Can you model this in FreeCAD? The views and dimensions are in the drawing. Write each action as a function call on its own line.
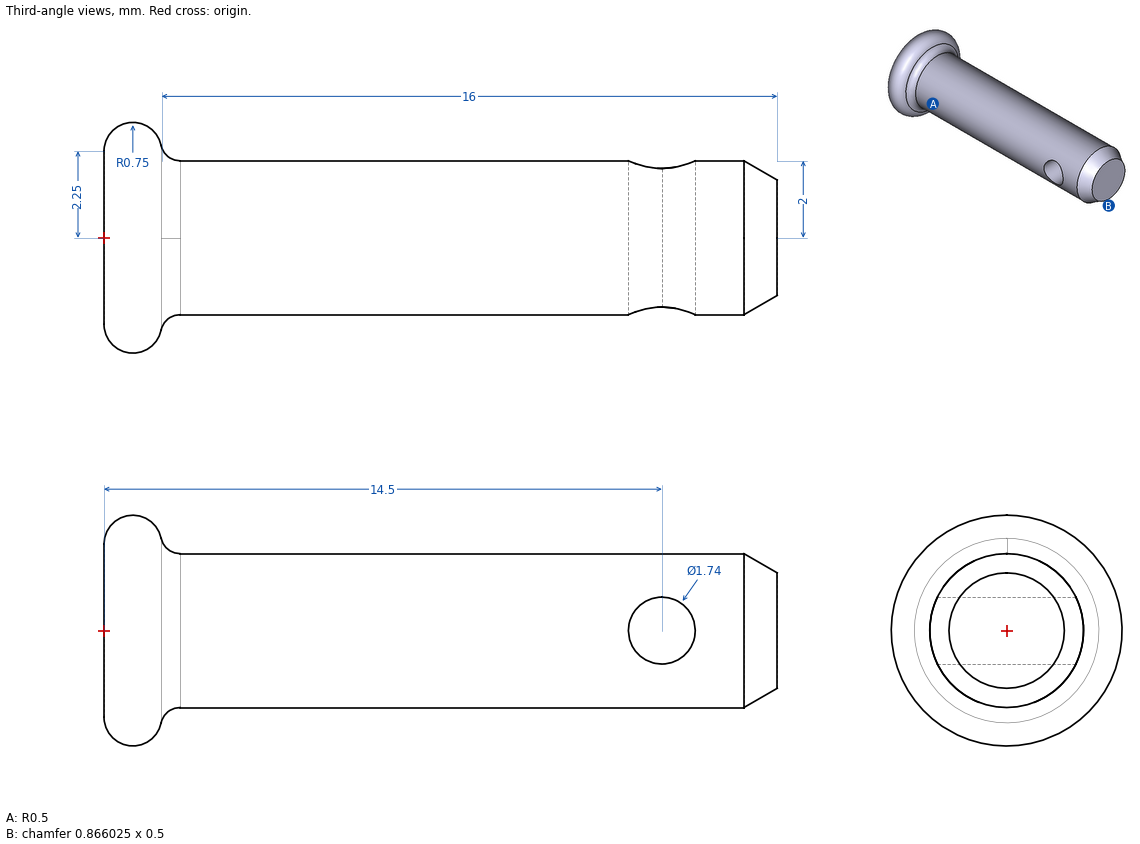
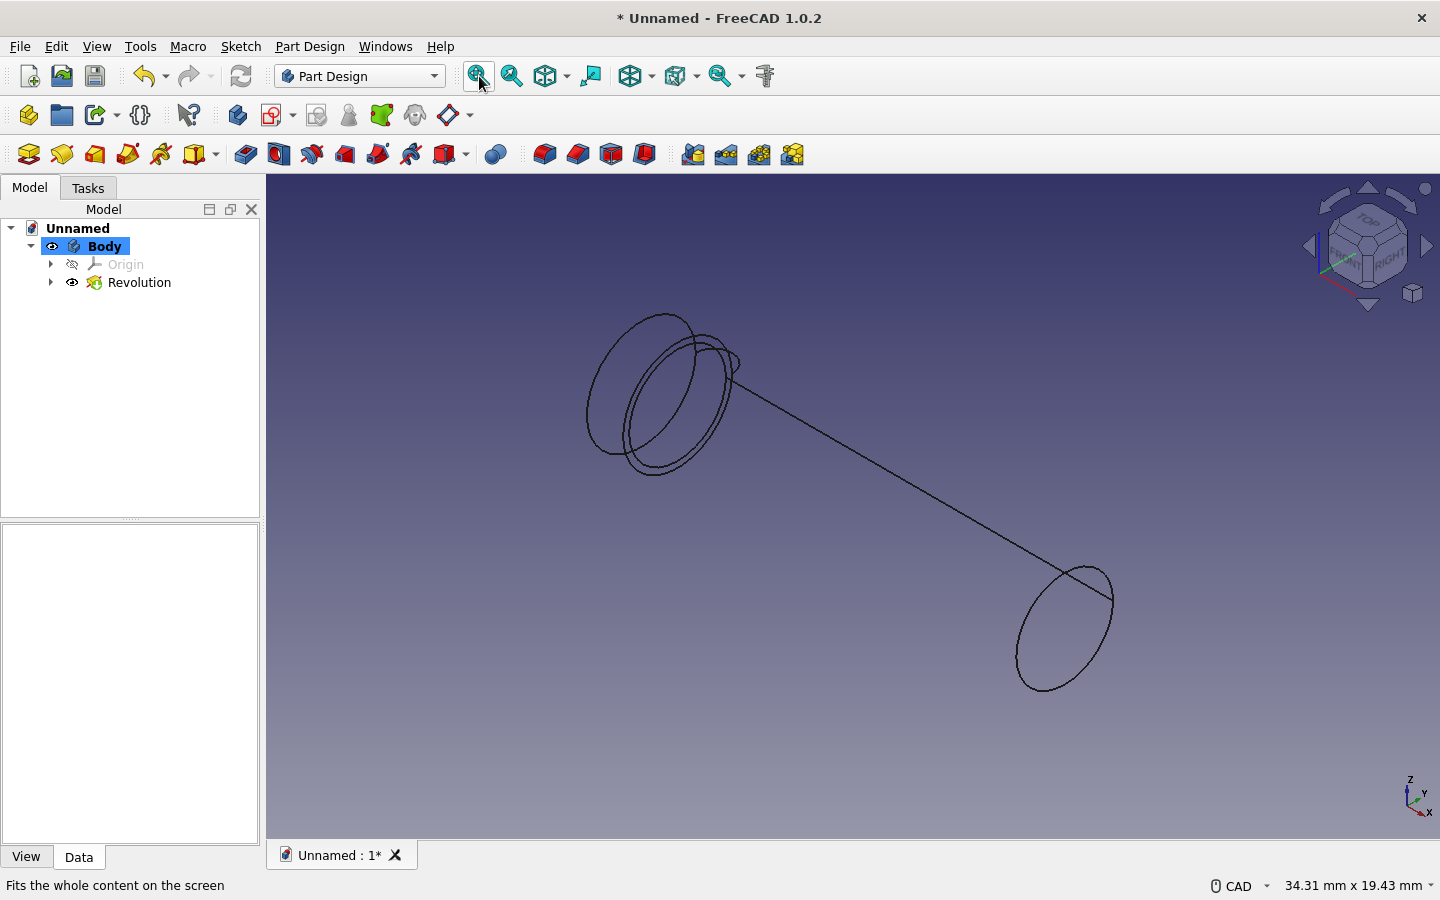
click(638, 460)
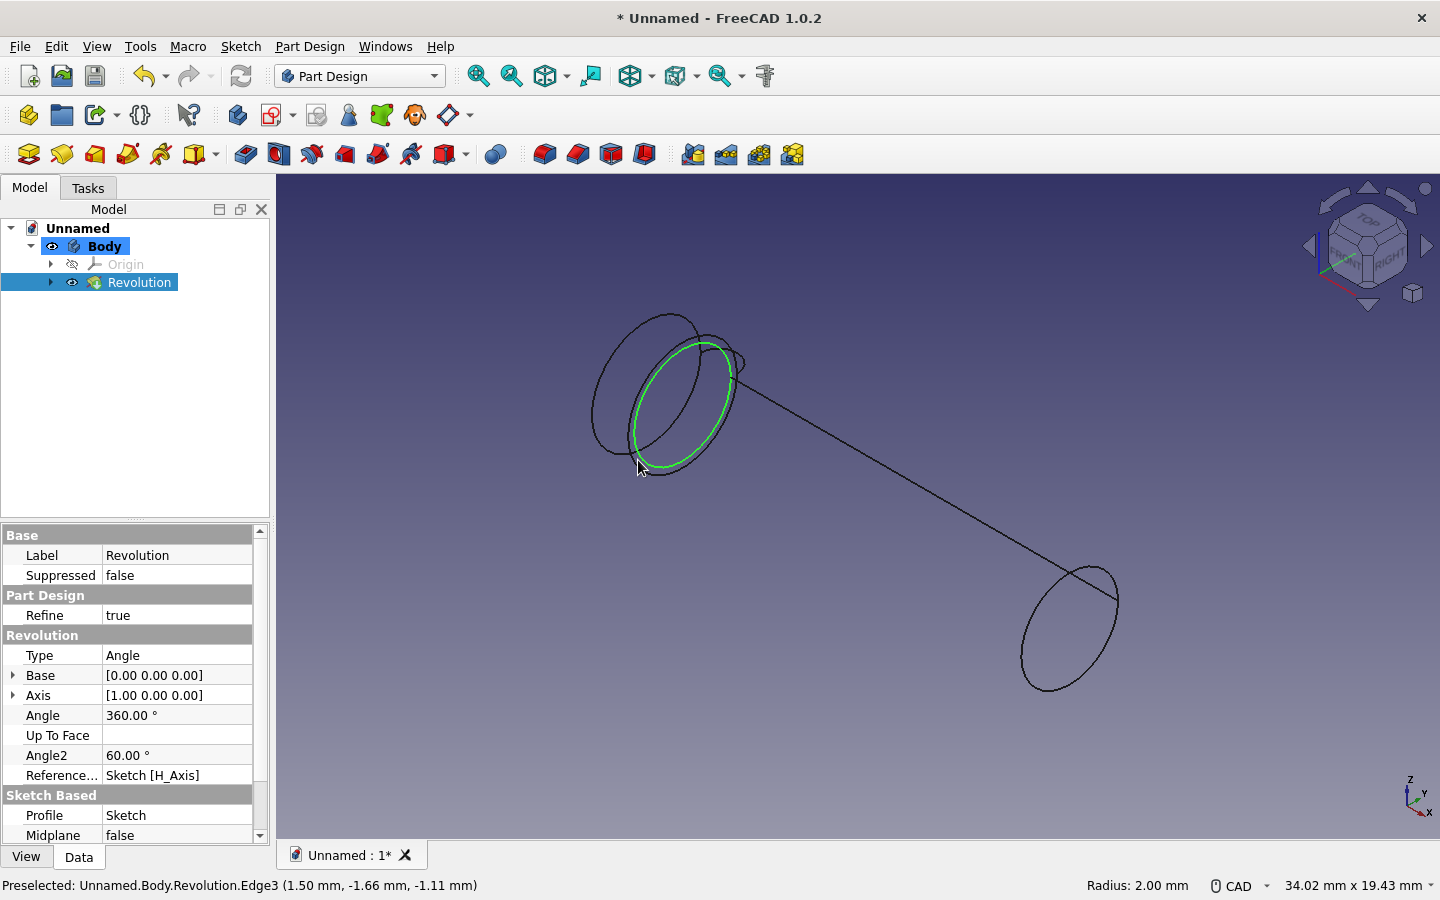
key(v)
key(1)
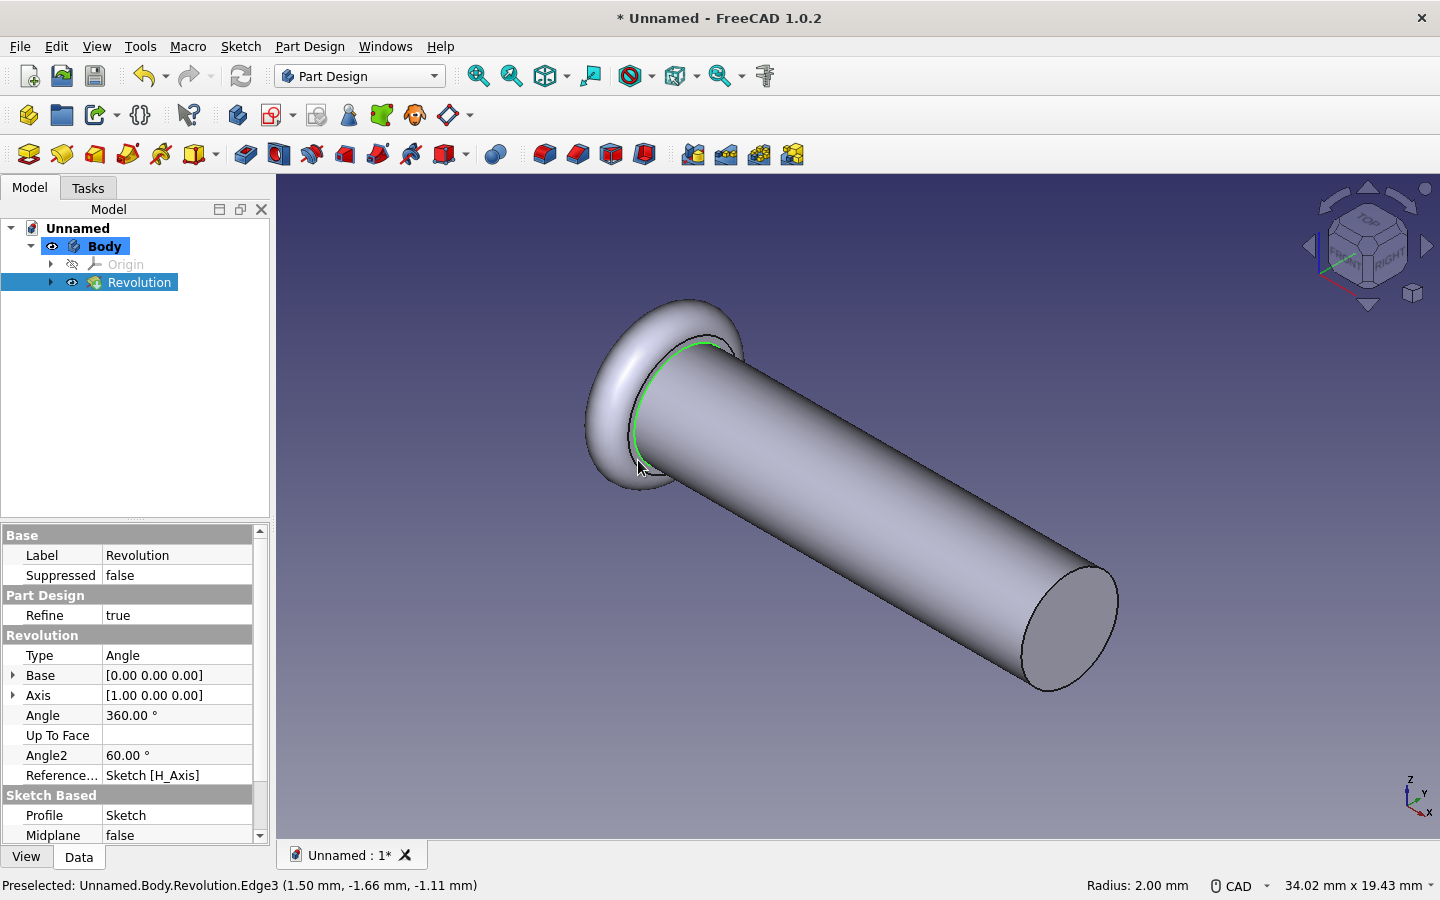
click(545, 154)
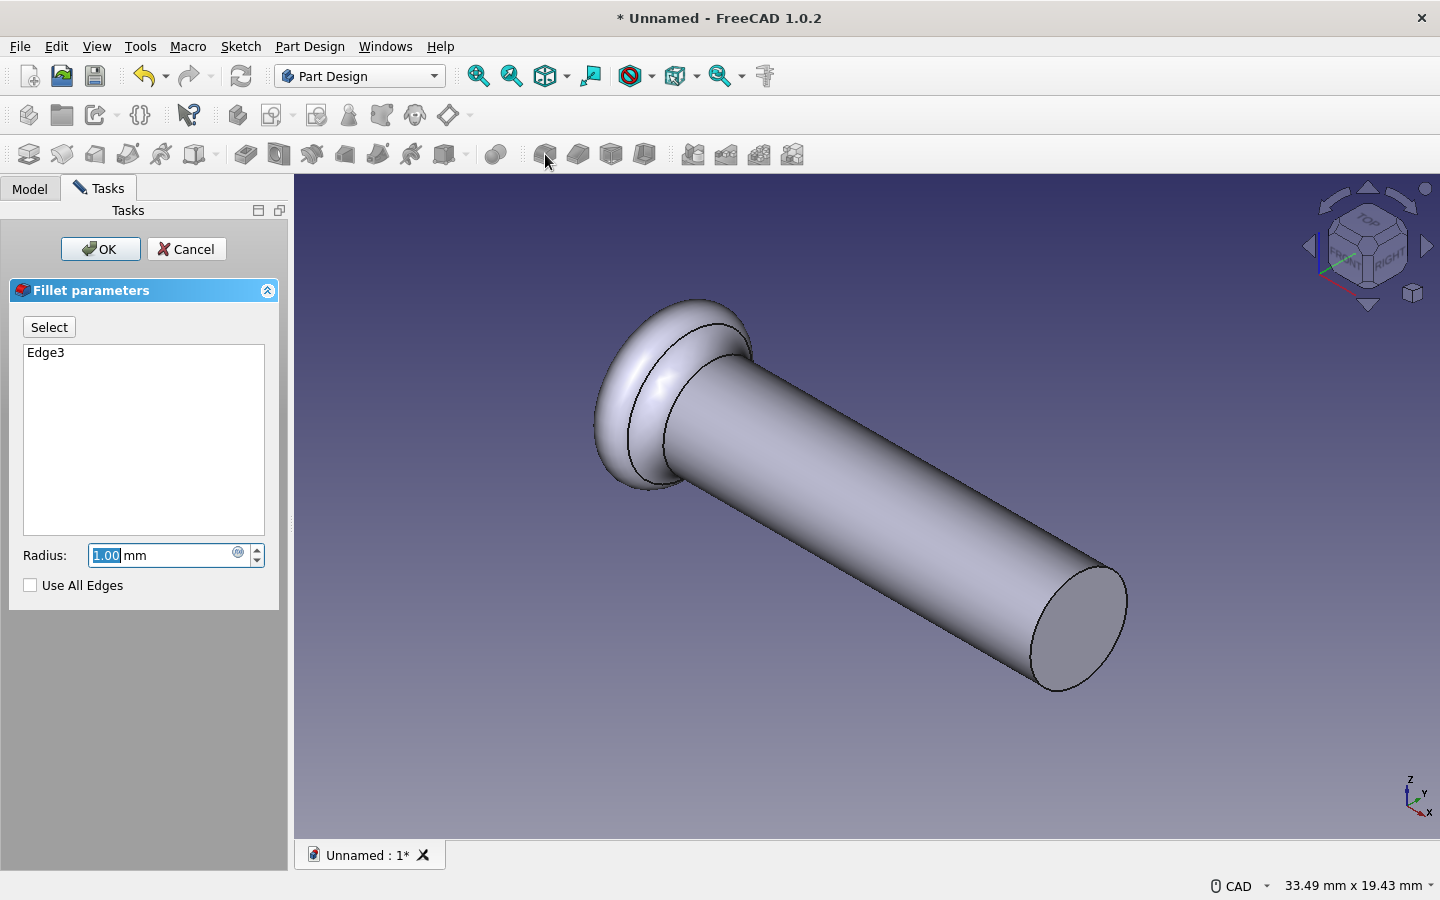
text(0.5)
key(Tab)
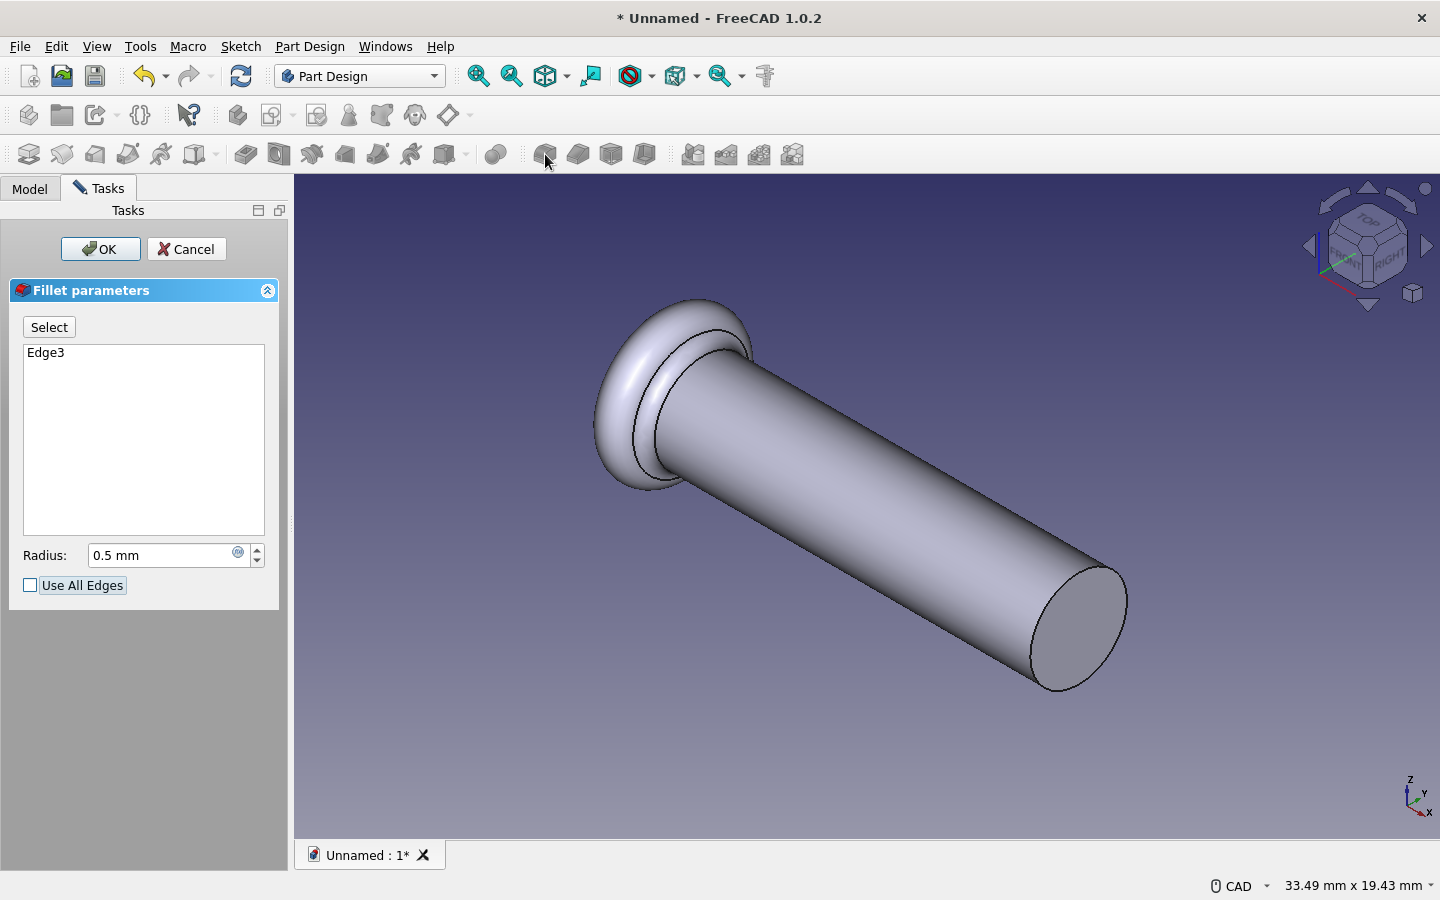
click(101, 249)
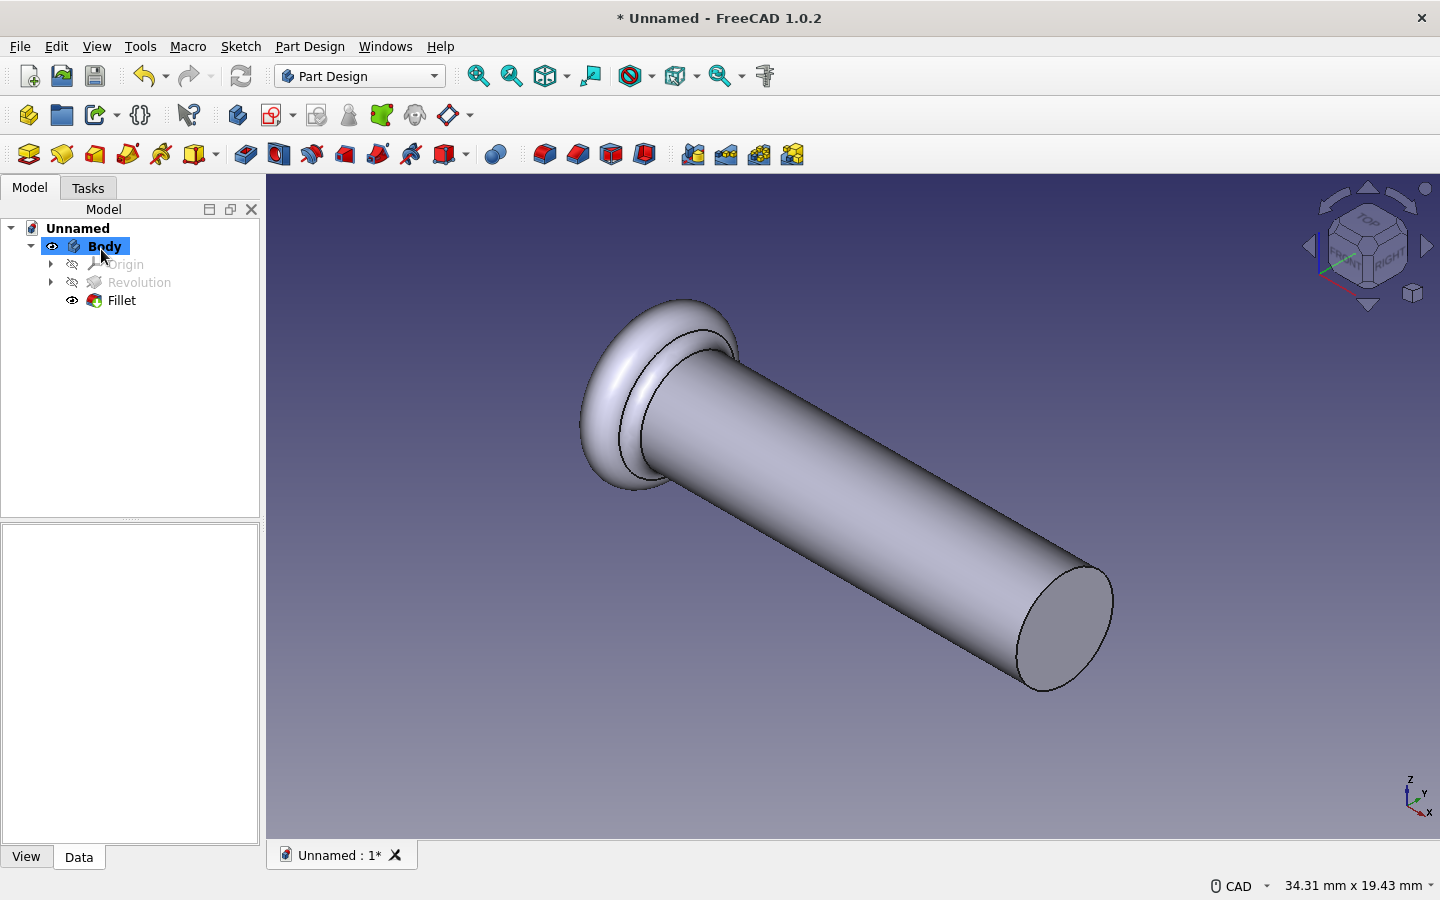
click(1016, 656)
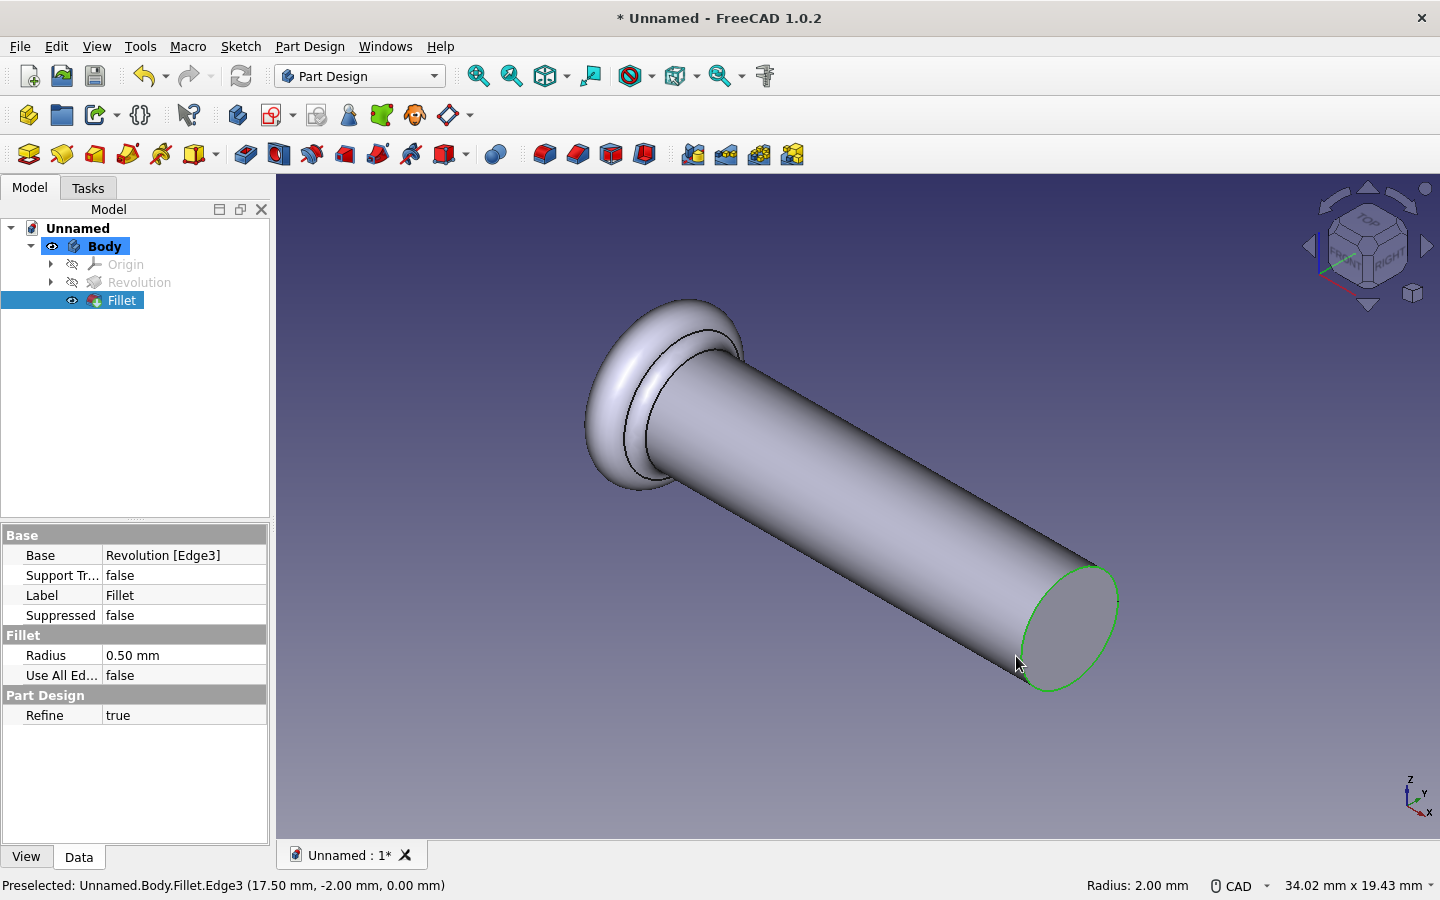
click(578, 154)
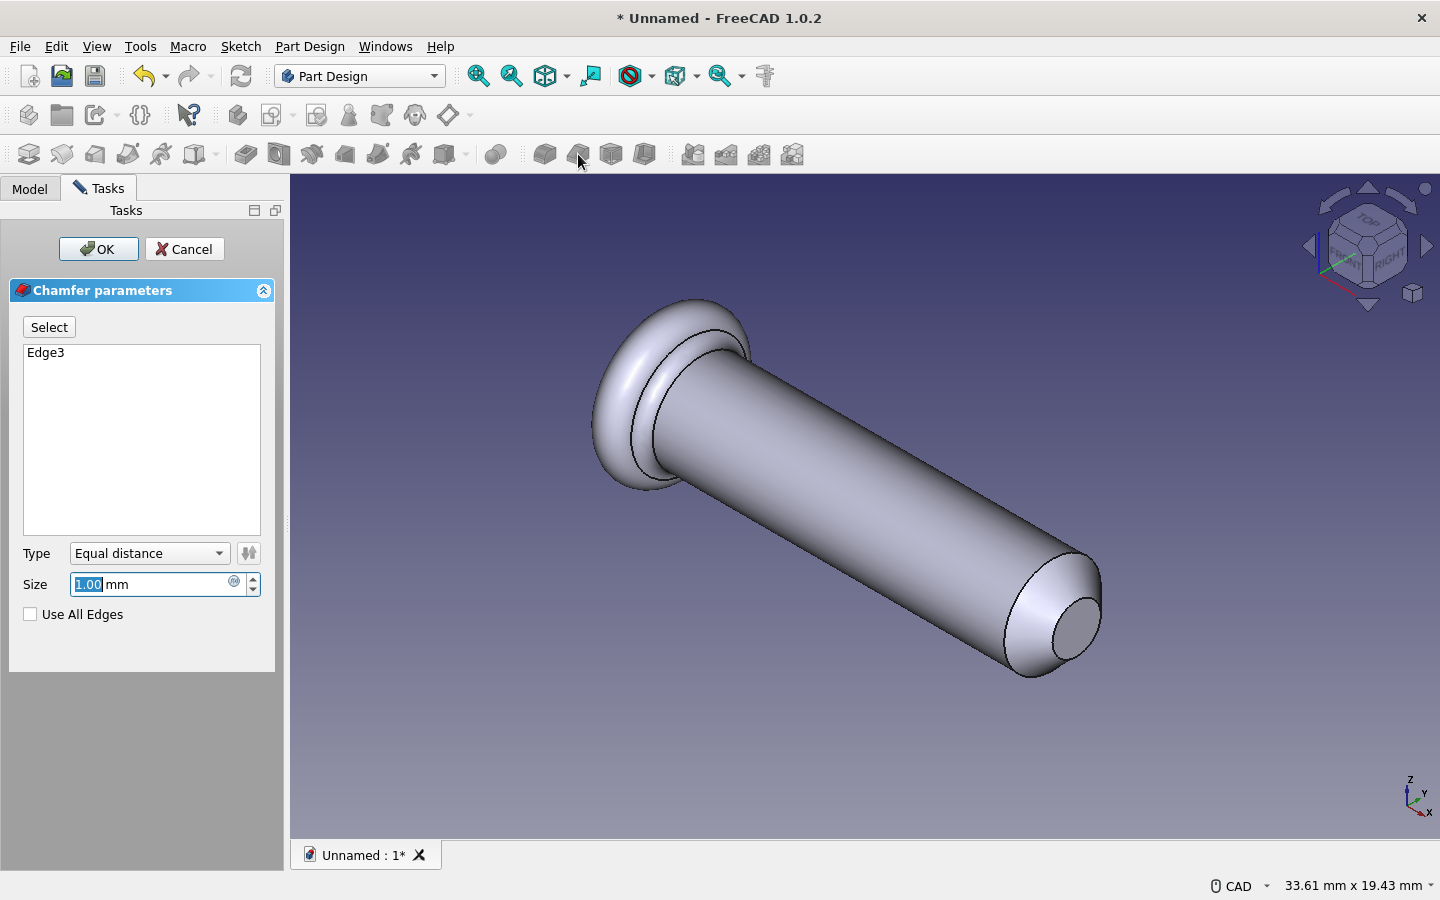
text(0.866025)
key(Tab)